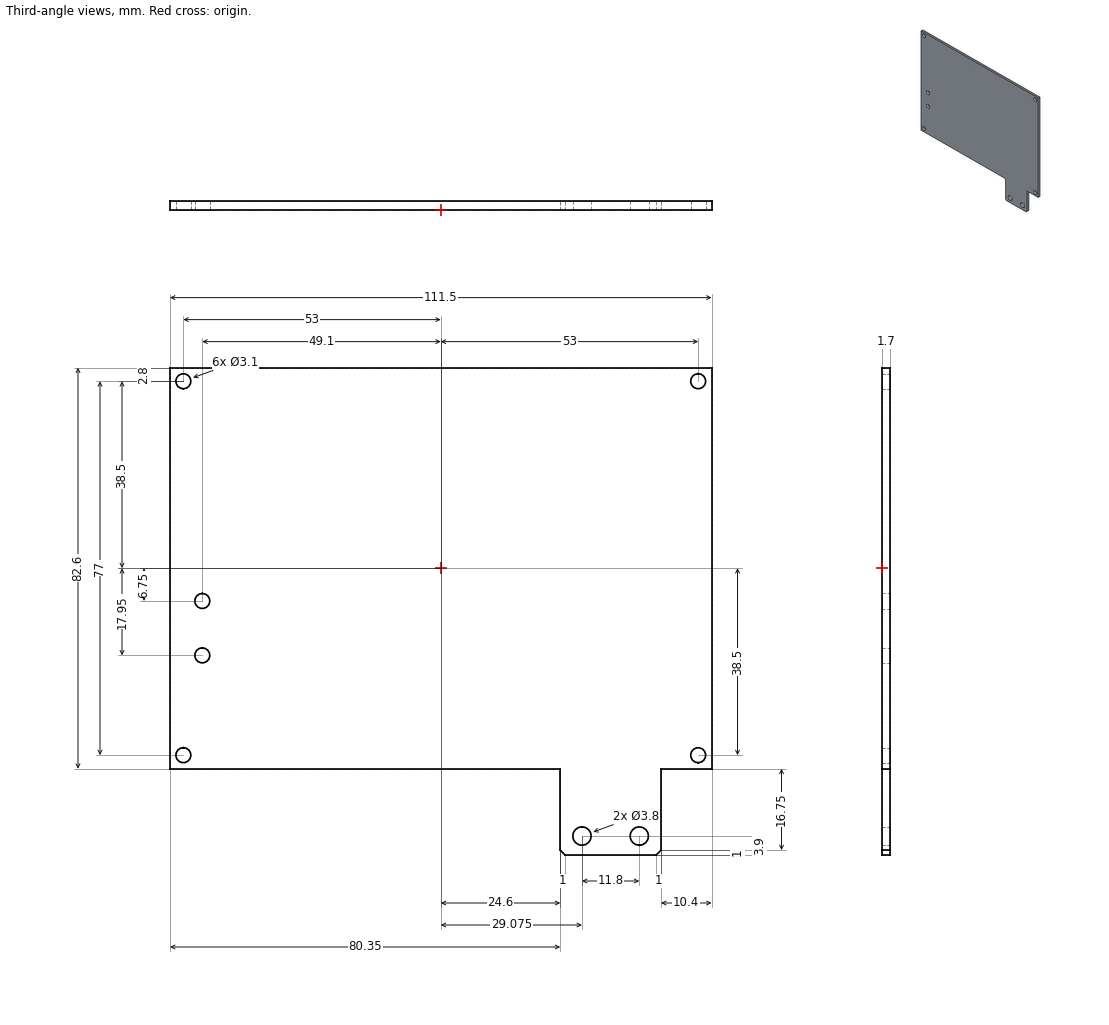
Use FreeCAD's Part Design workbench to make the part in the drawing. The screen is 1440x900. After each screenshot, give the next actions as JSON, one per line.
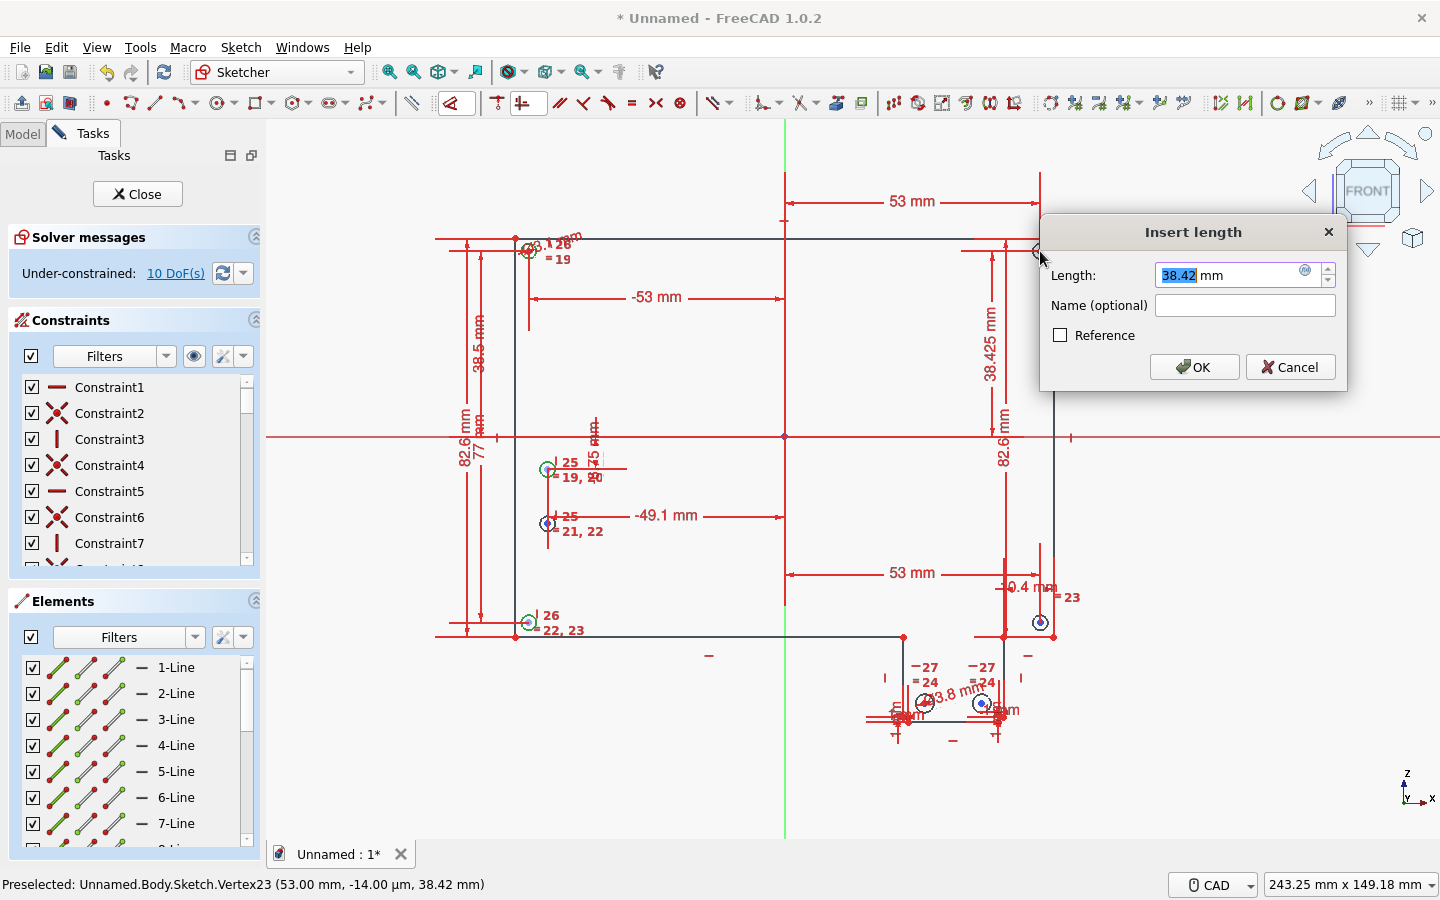
{"action": "type", "text": "38.5"}
{"action": "key", "text": "Return"}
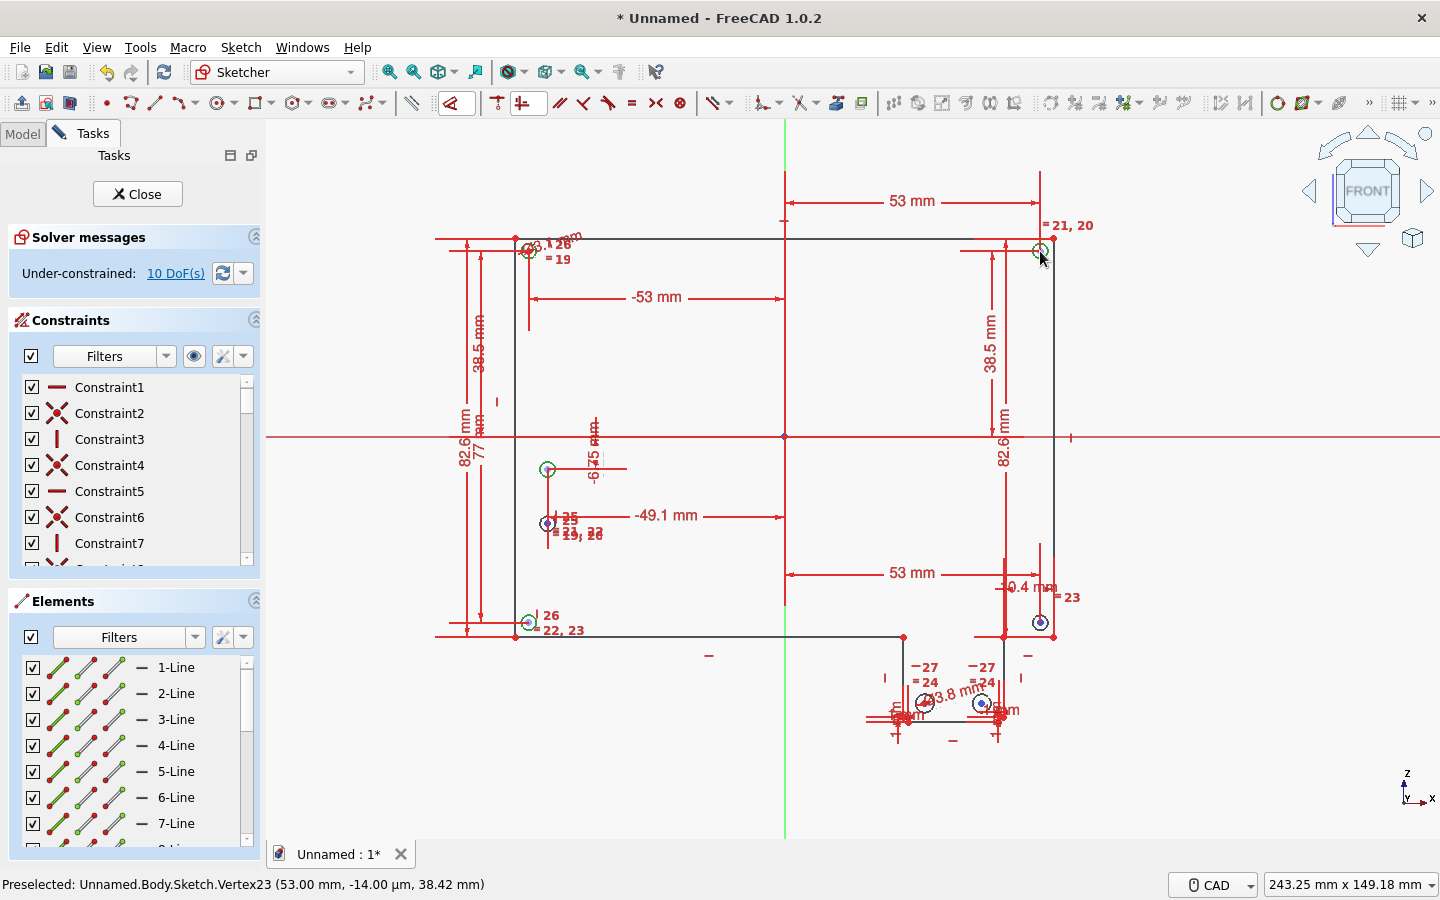
{"action": "left_click", "coordinate": [1040, 623]}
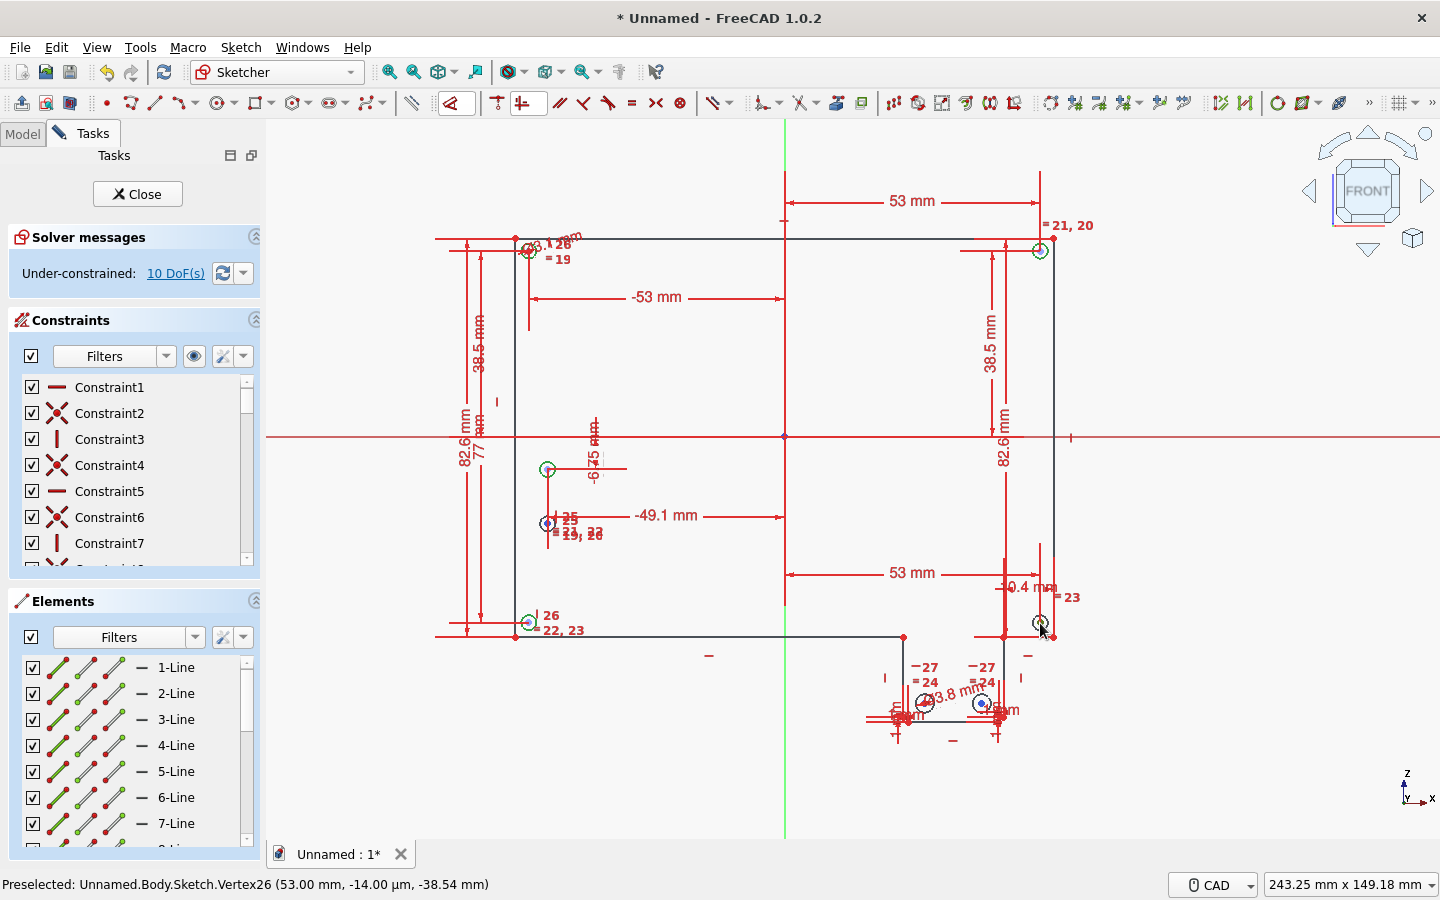
{"action": "key", "text": "i"}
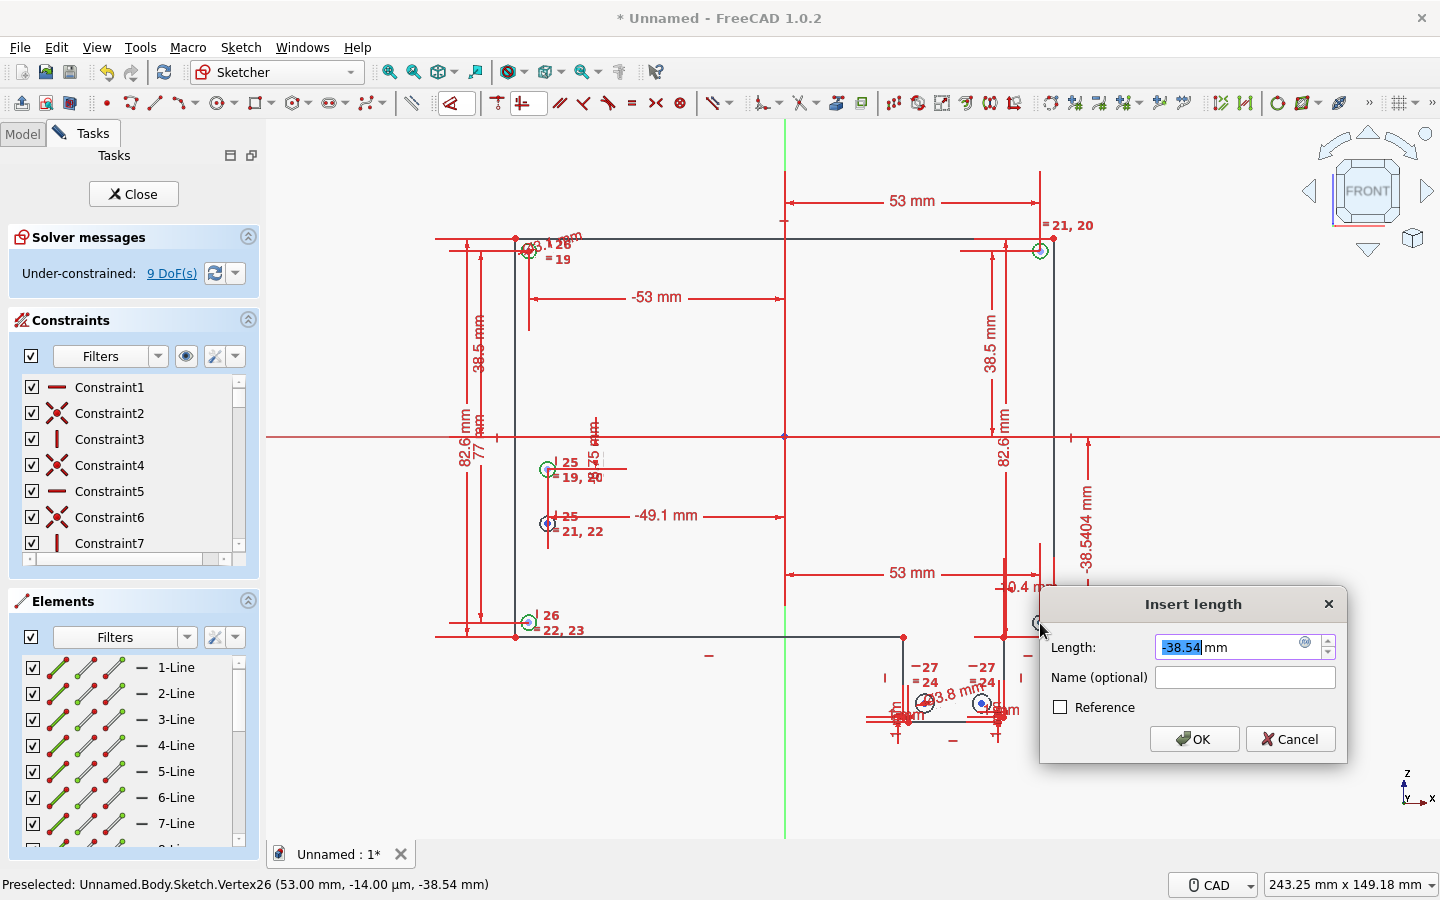
{"action": "type", "text": "-38.5"}
{"action": "key", "text": "Return"}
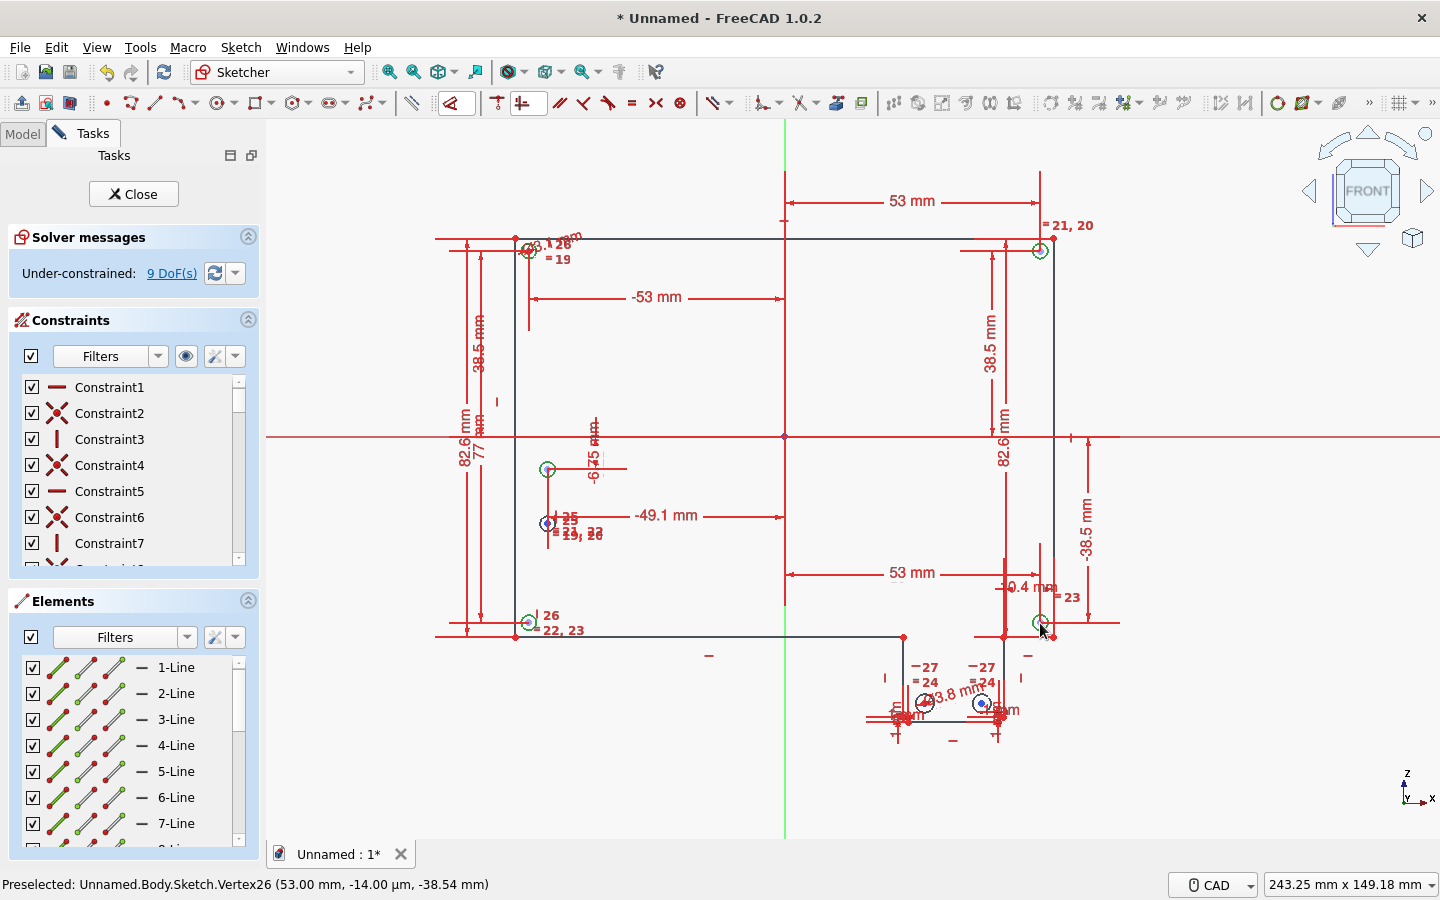
{"action": "scroll", "coordinate": [515, 239], "scroll_direction": "up", "scroll_amount": 6}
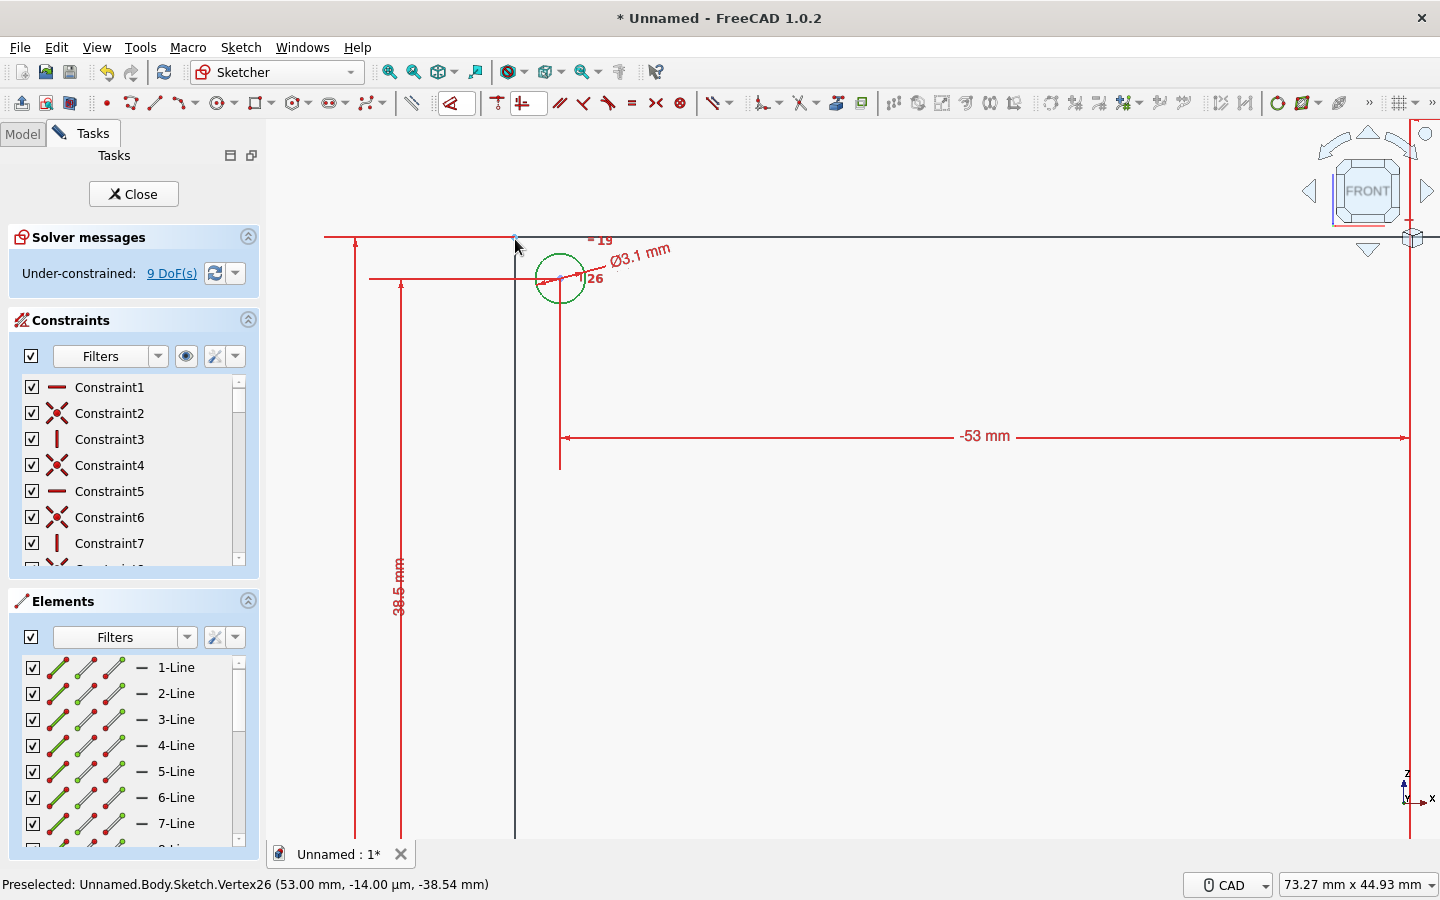
{"action": "left_click", "coordinate": [515, 237]}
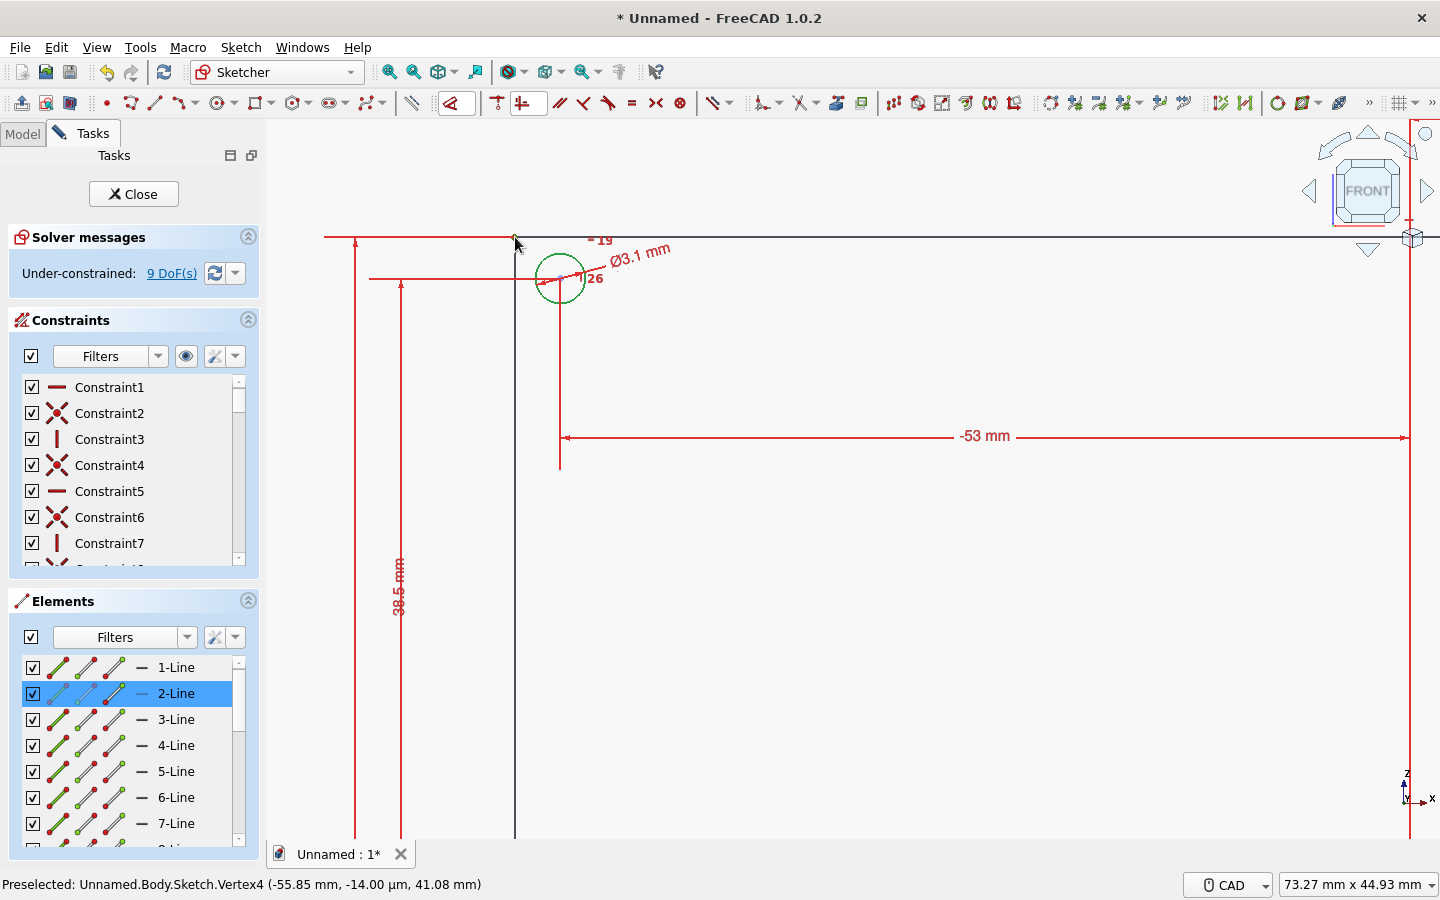
{"action": "left_click", "coordinate": [560, 279]}